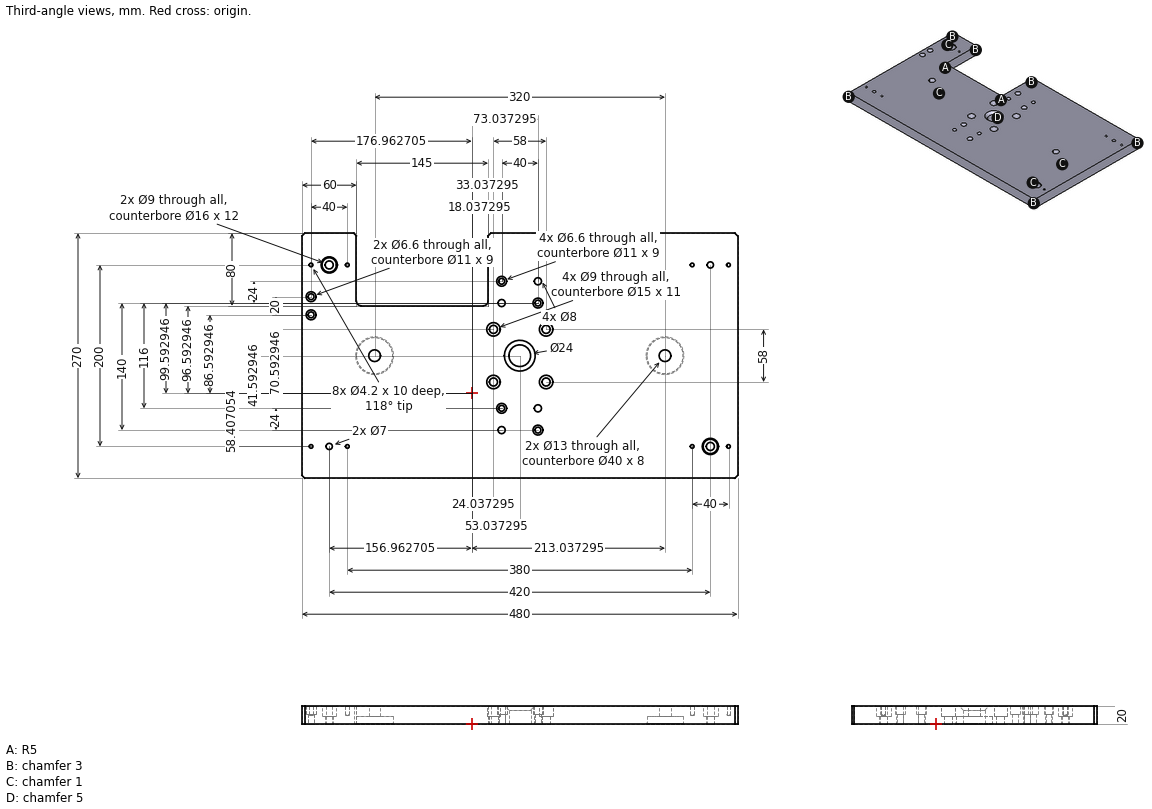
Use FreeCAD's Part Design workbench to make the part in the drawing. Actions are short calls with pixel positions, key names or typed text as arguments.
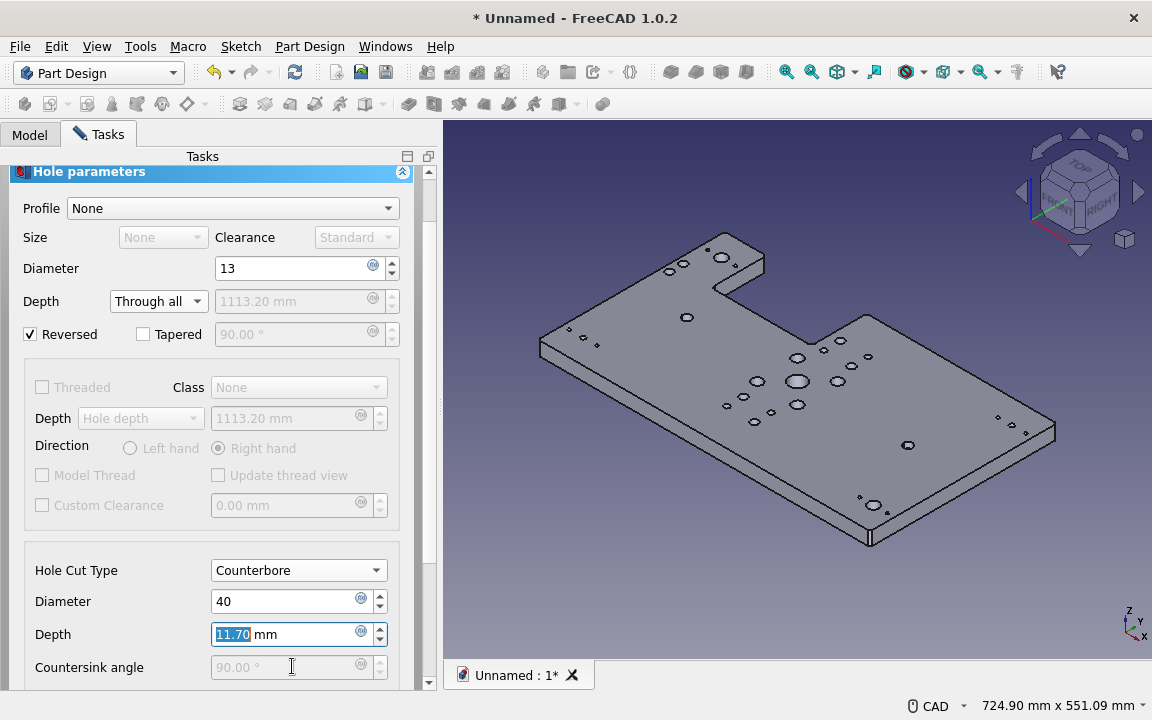
text(8)
key(Tab)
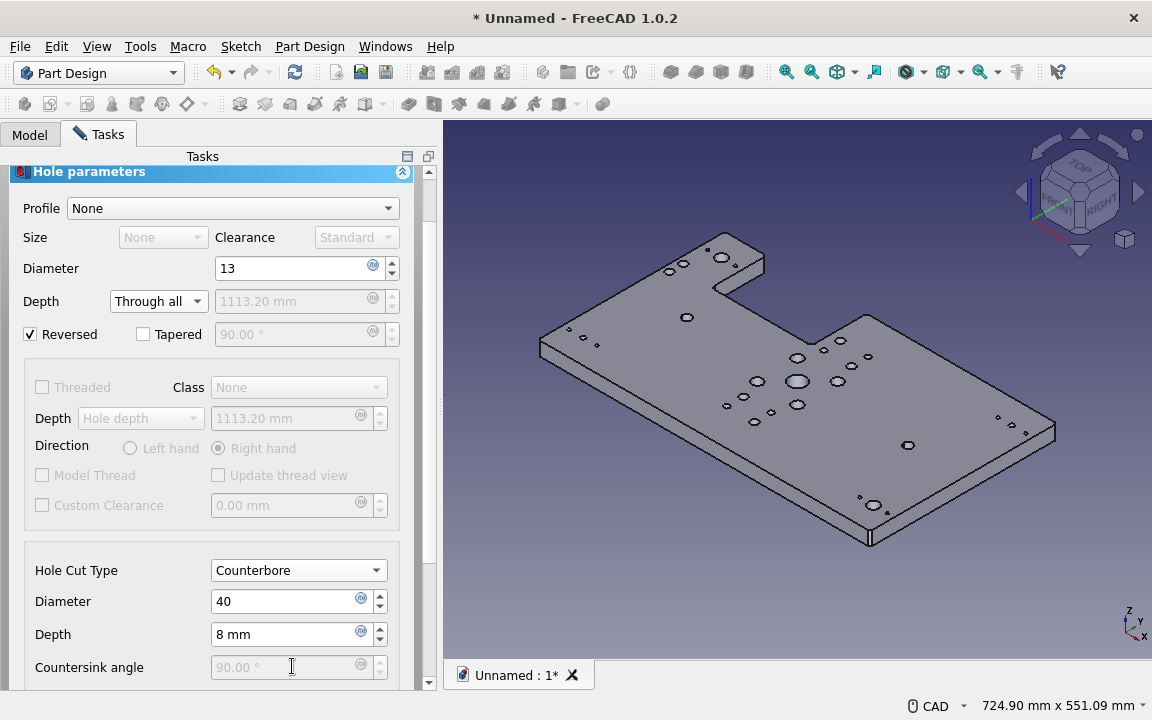
scroll(429, 428, up, 2)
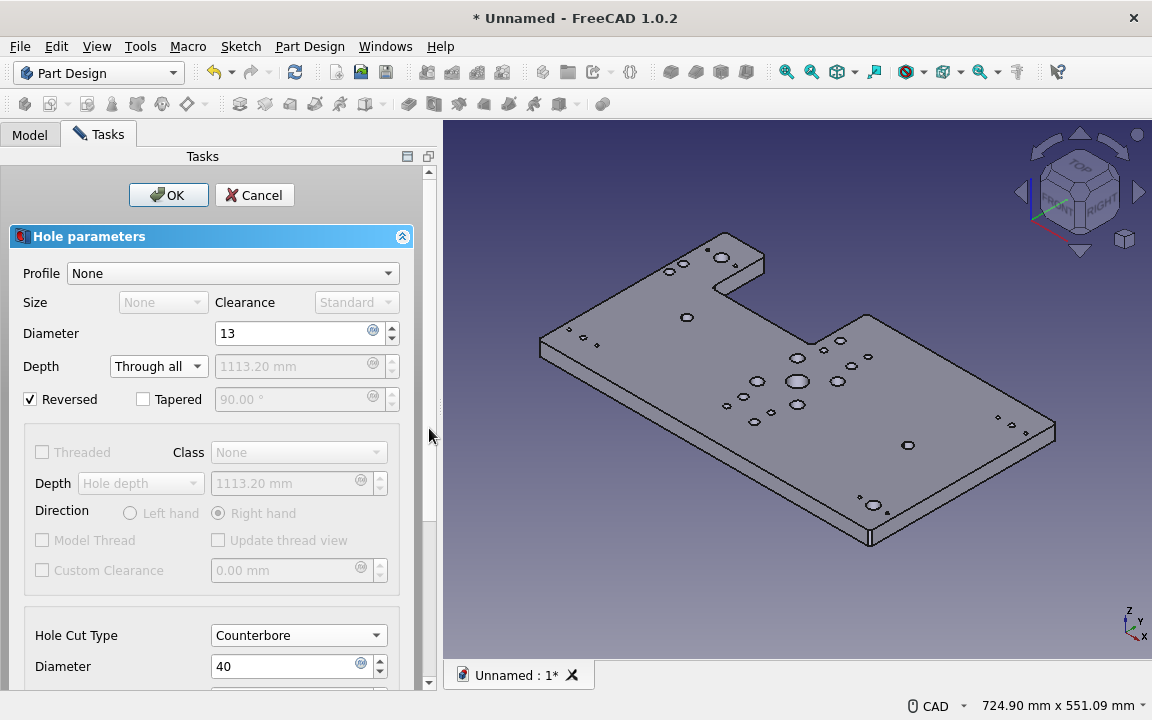
click(169, 195)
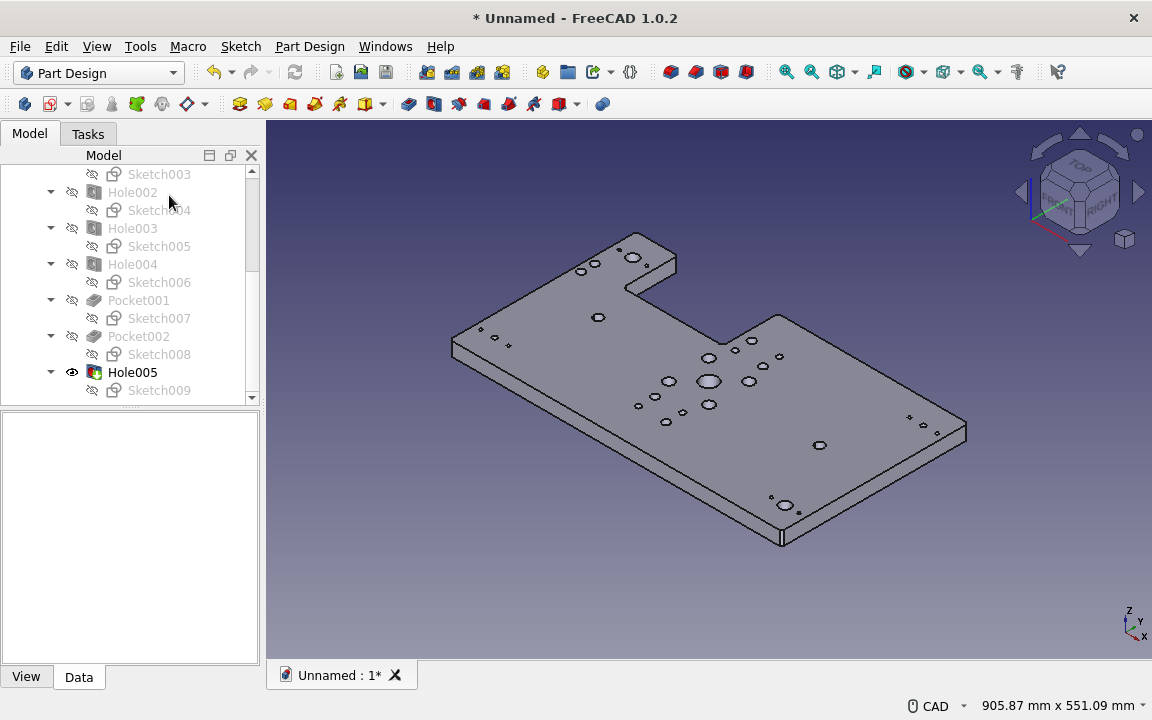
click(780, 501)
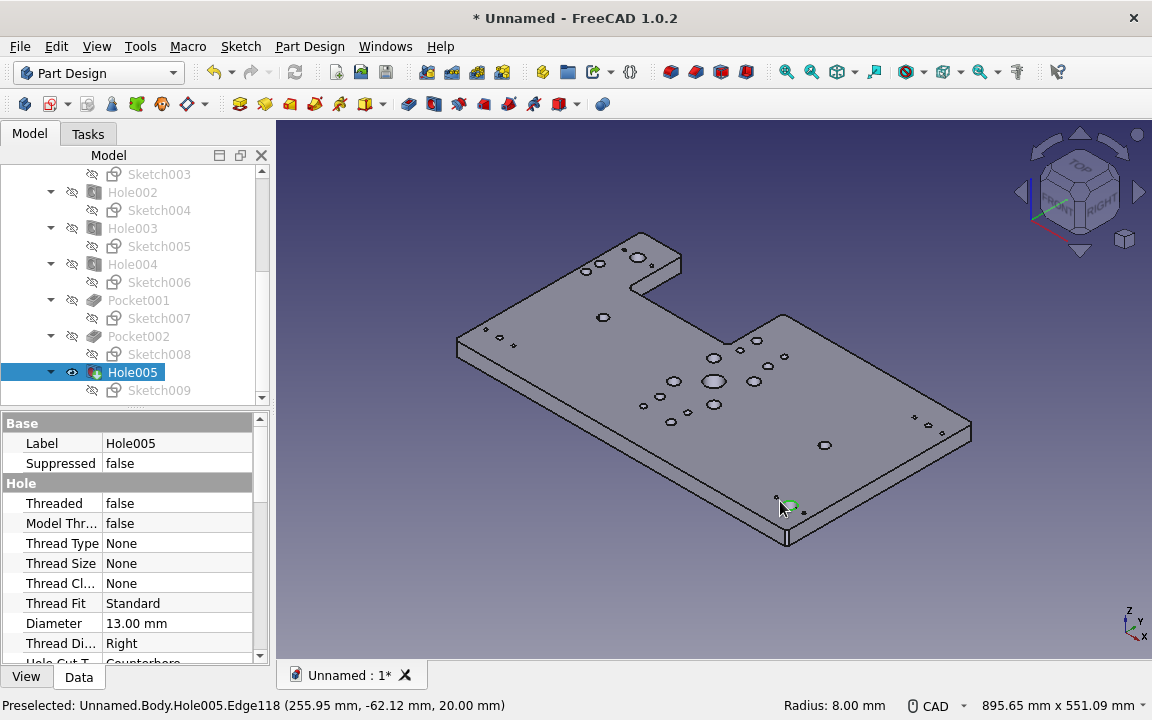
click(632, 254, ctrl)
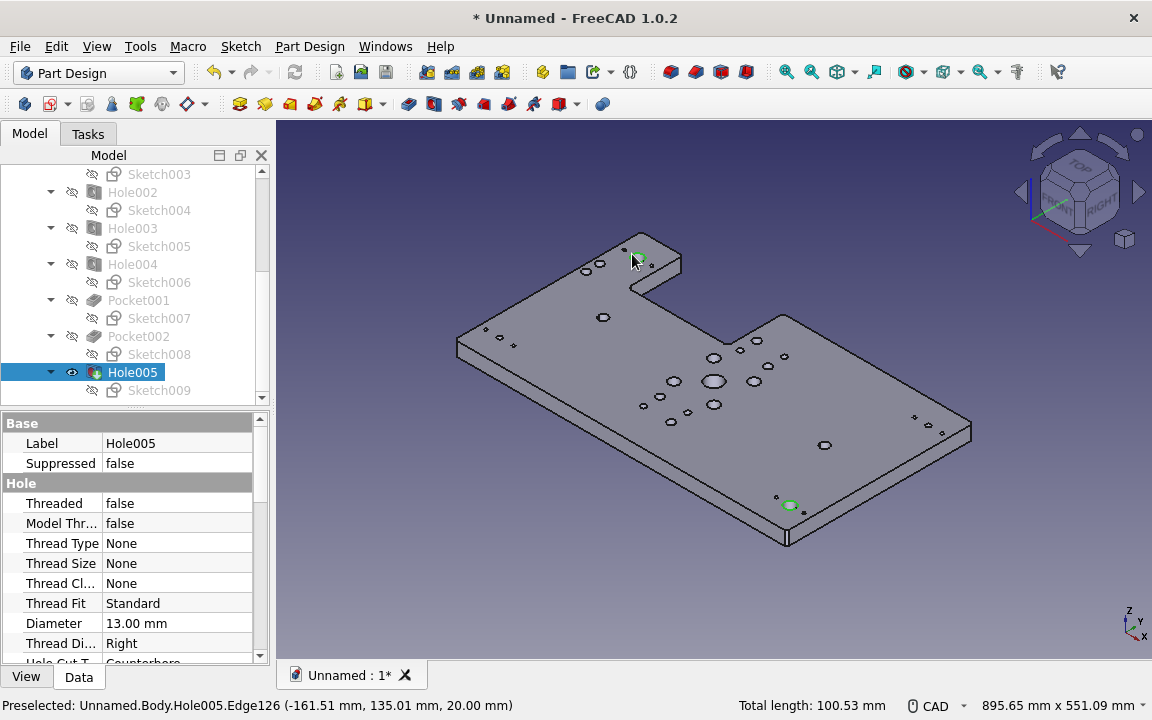
key(2)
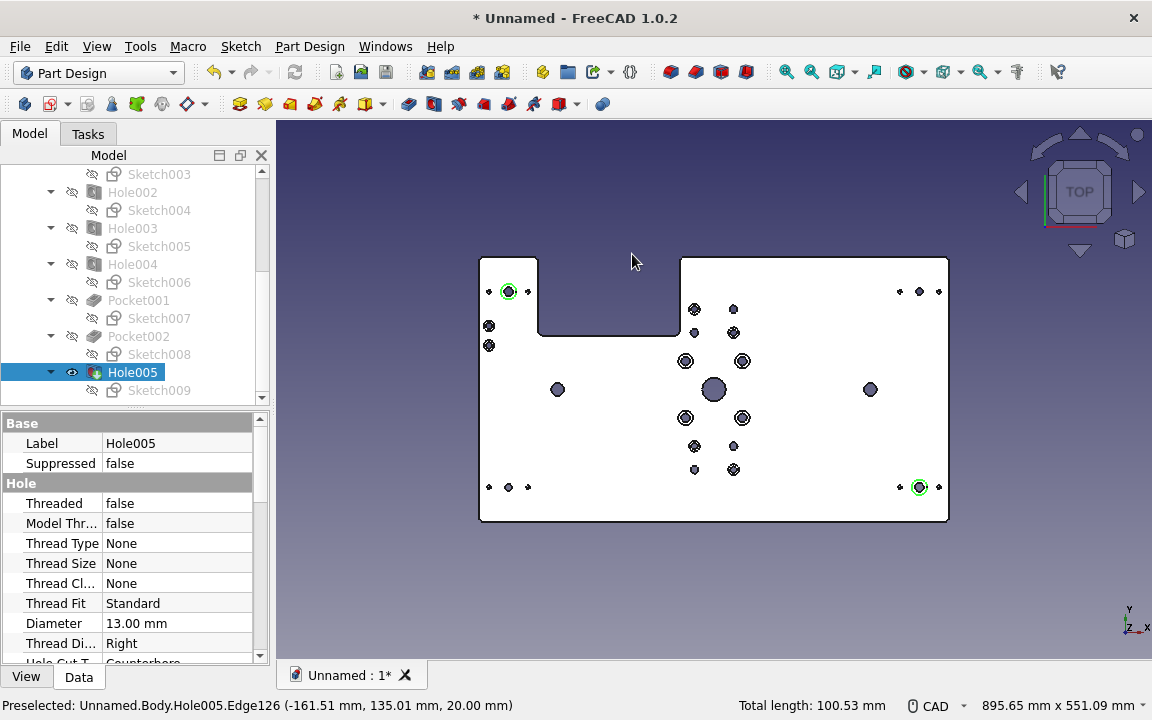
key(0)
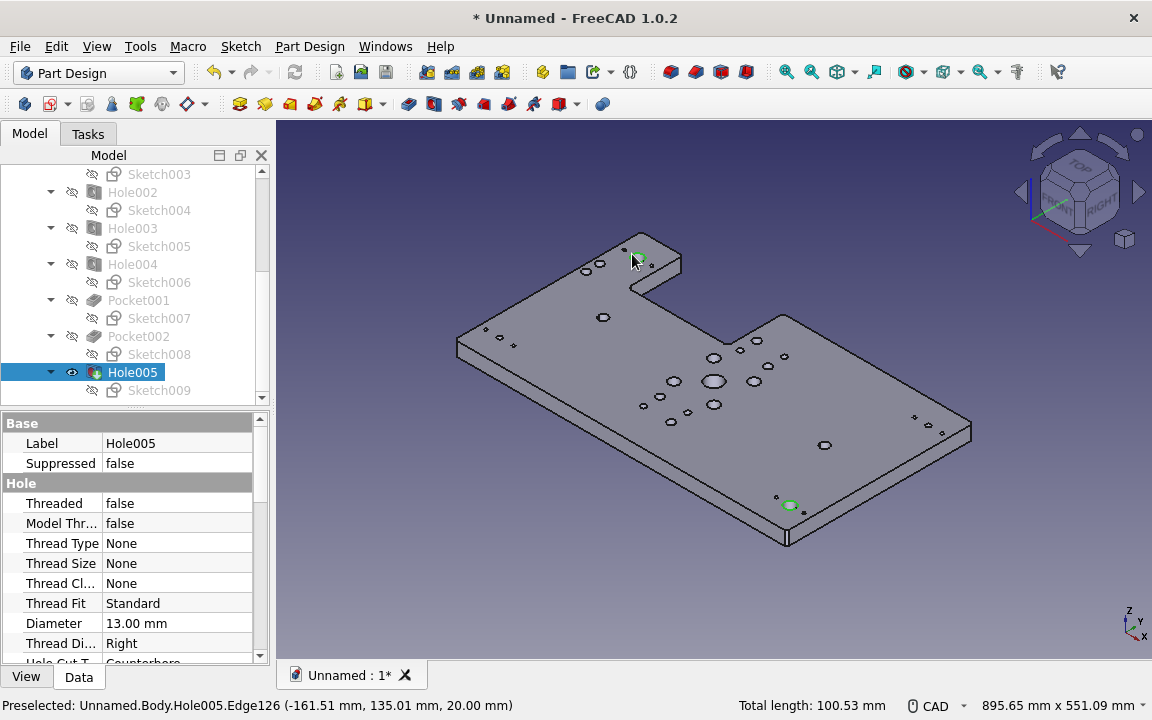
key(1)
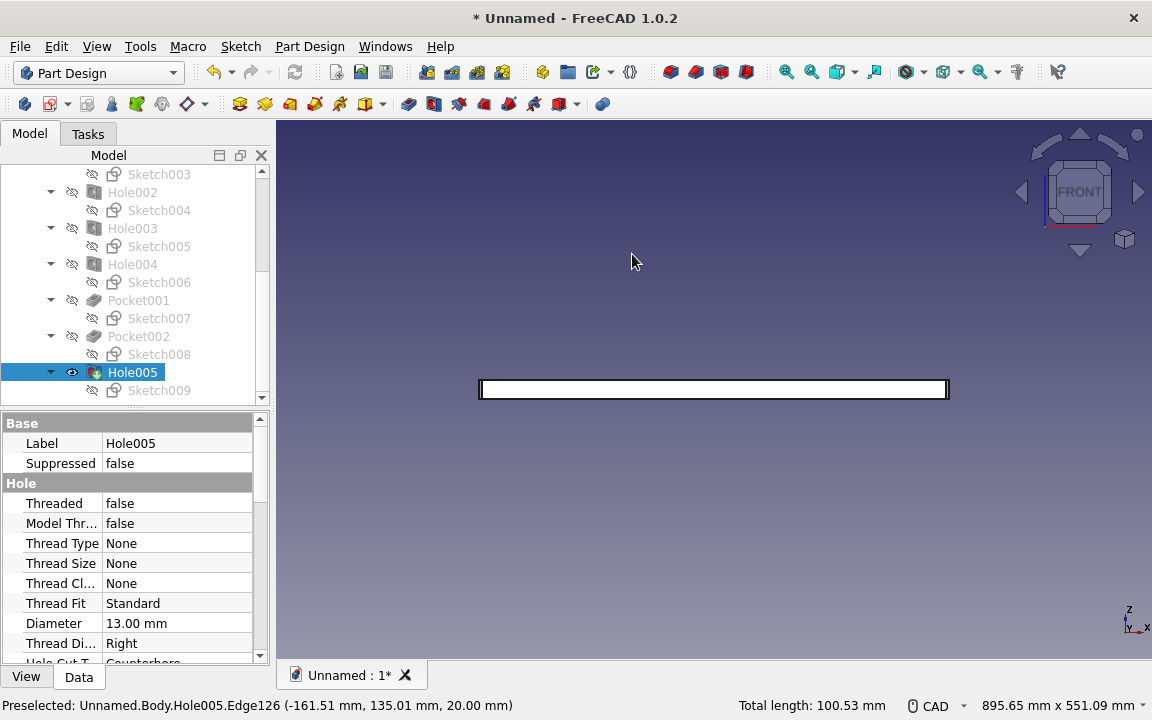
key(3)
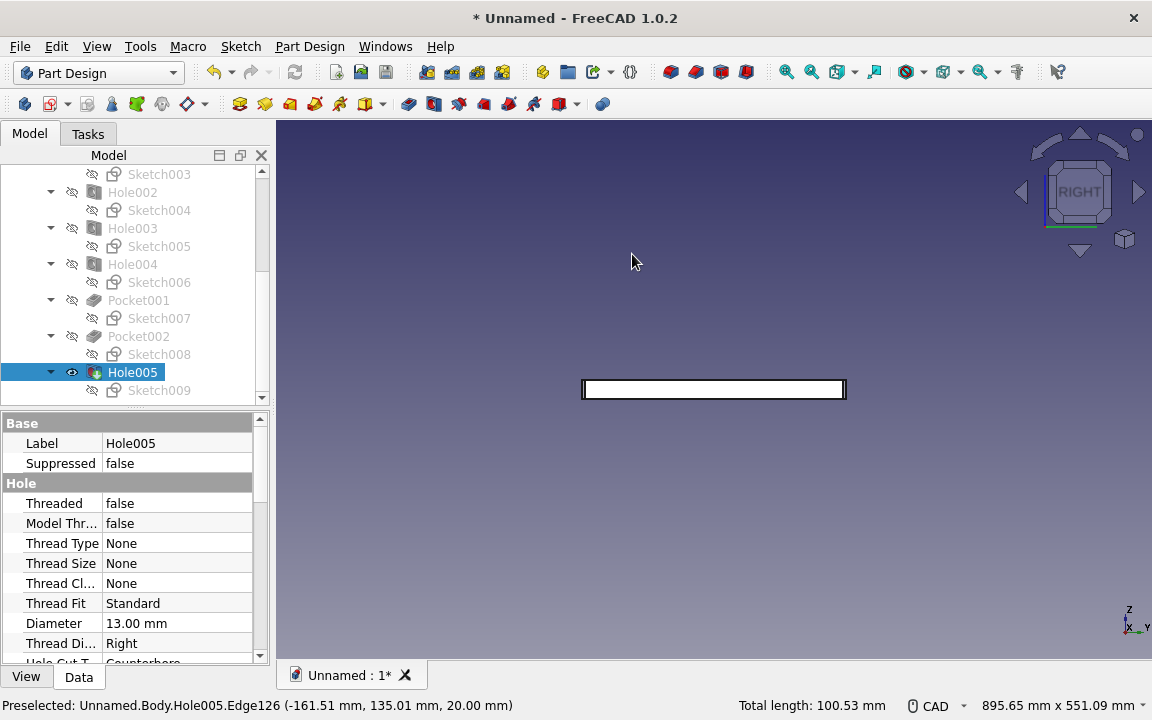
key(v)
key(f)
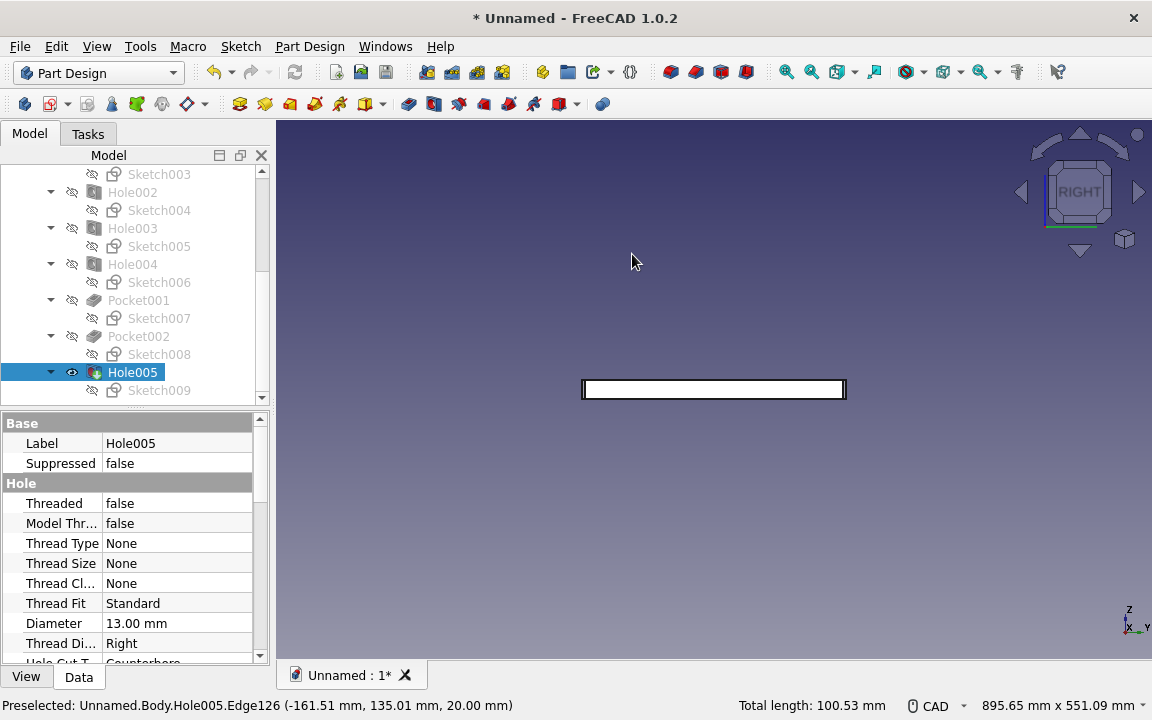
key(5)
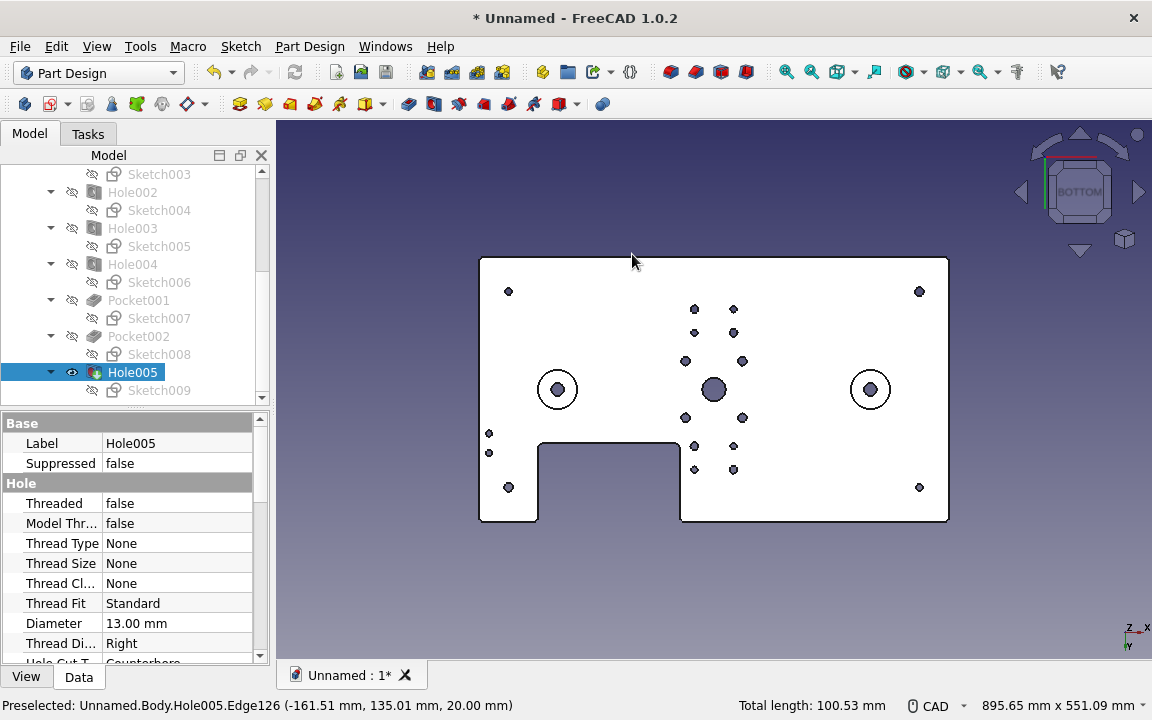
click(577, 388, ctrl)